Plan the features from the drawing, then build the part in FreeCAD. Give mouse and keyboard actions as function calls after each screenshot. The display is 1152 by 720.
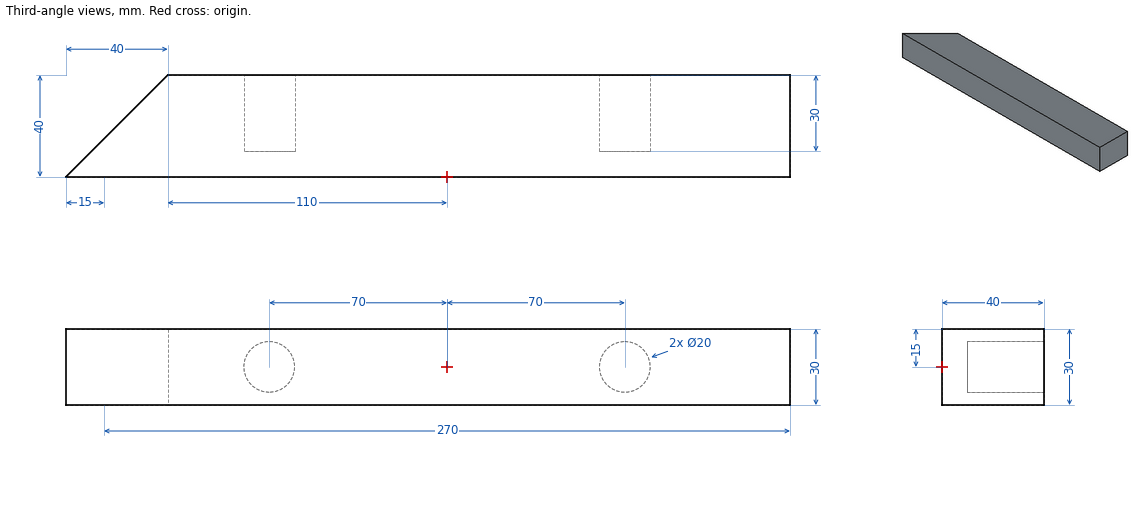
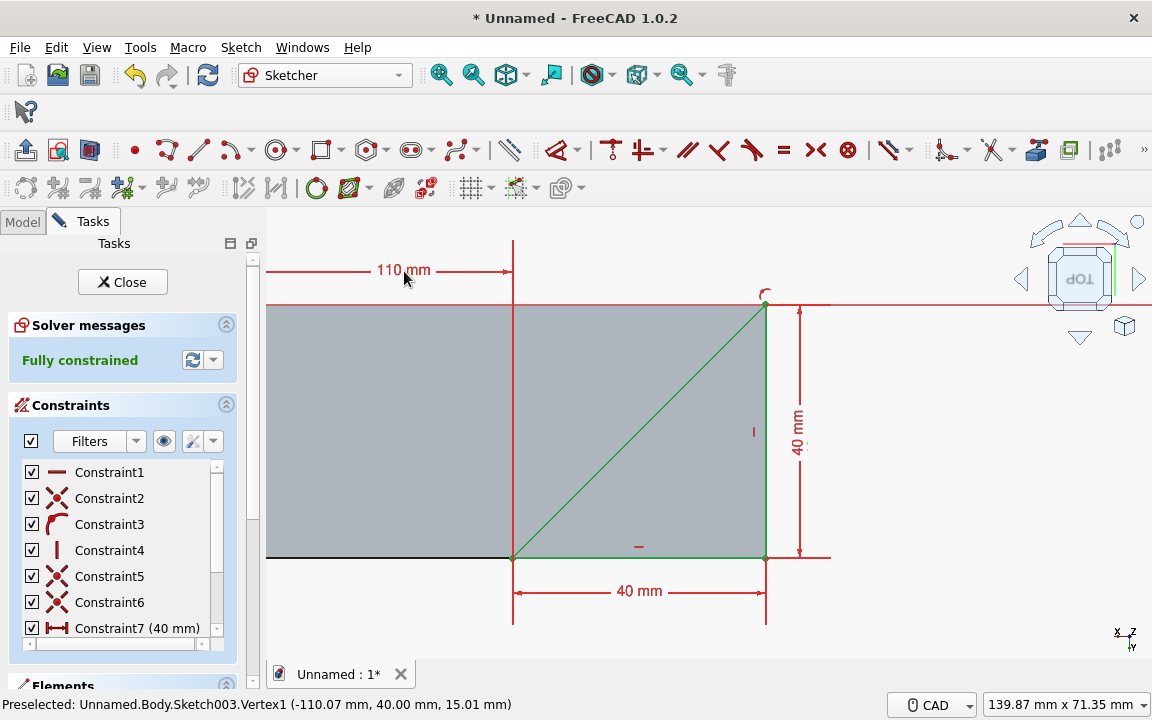
click(123, 282)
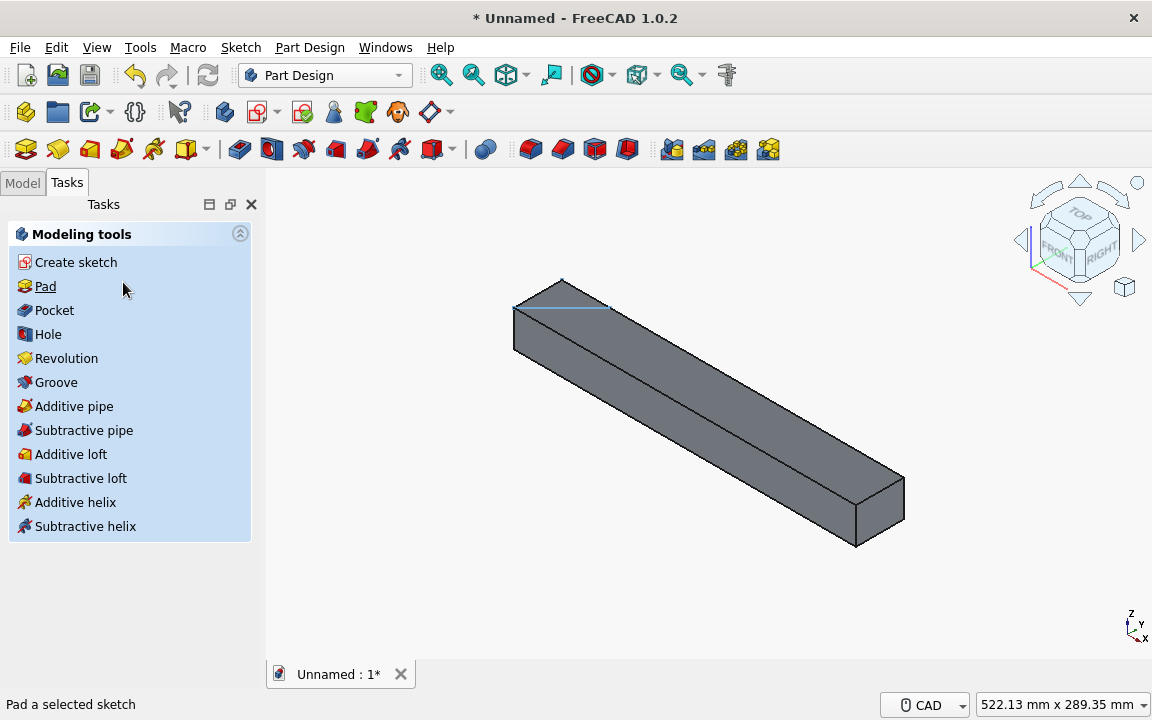
click(240, 150)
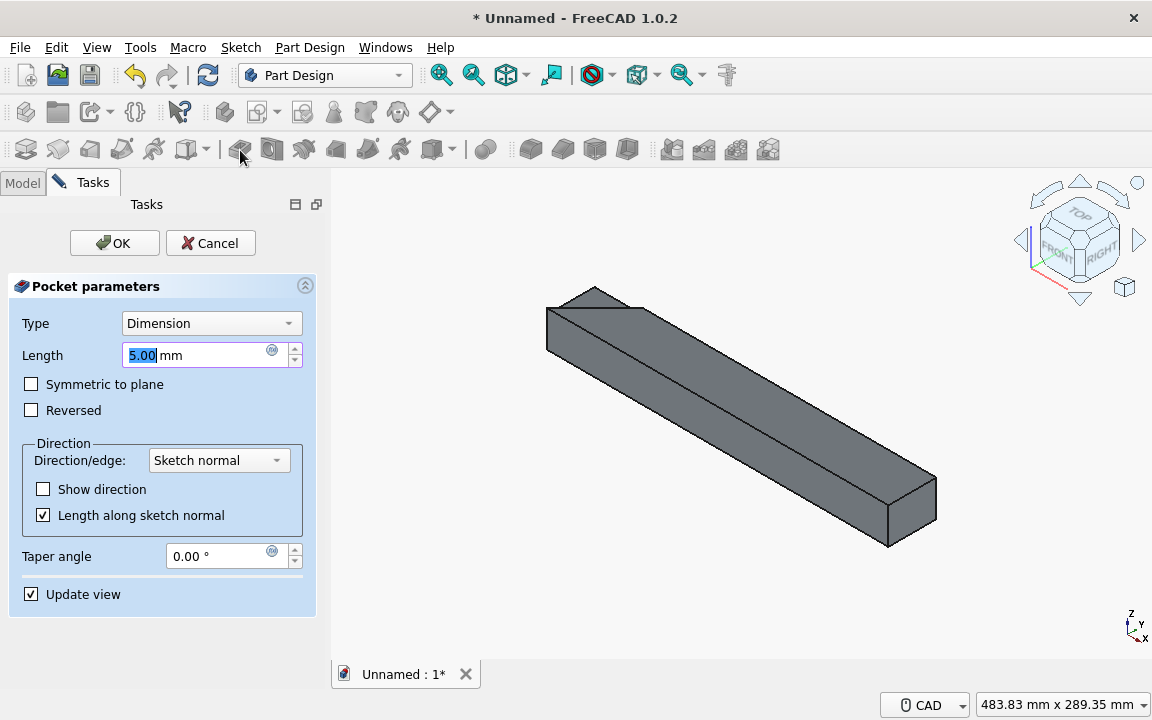
click(212, 324)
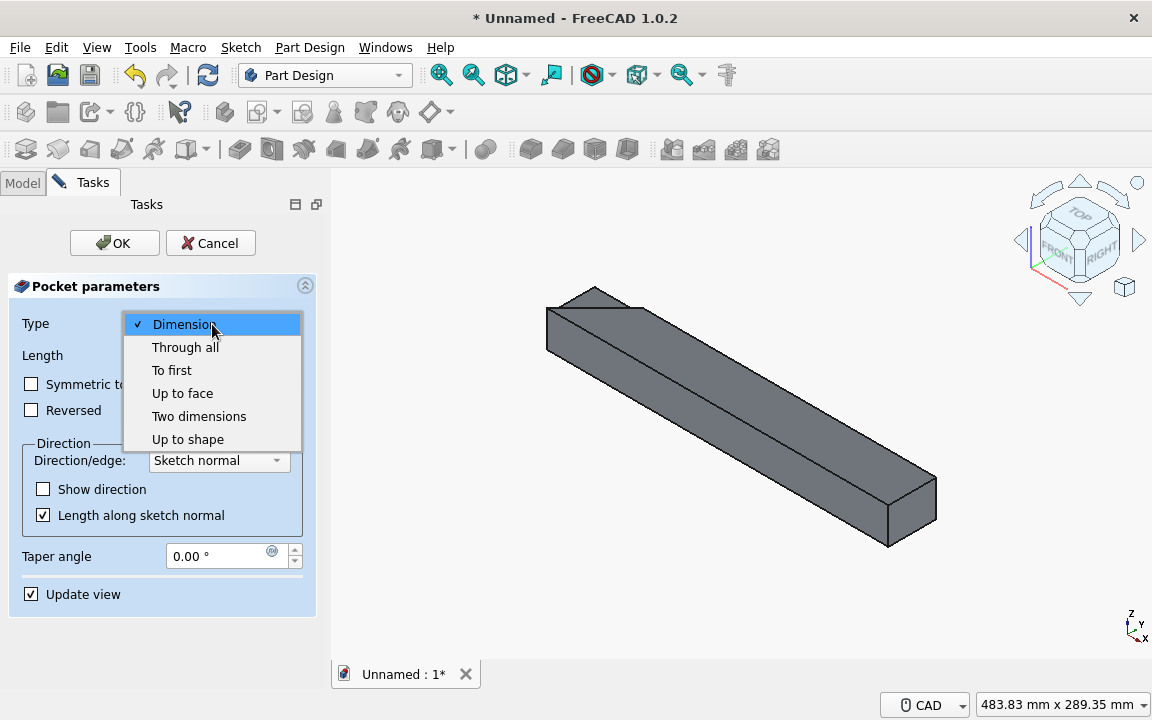
click(212, 348)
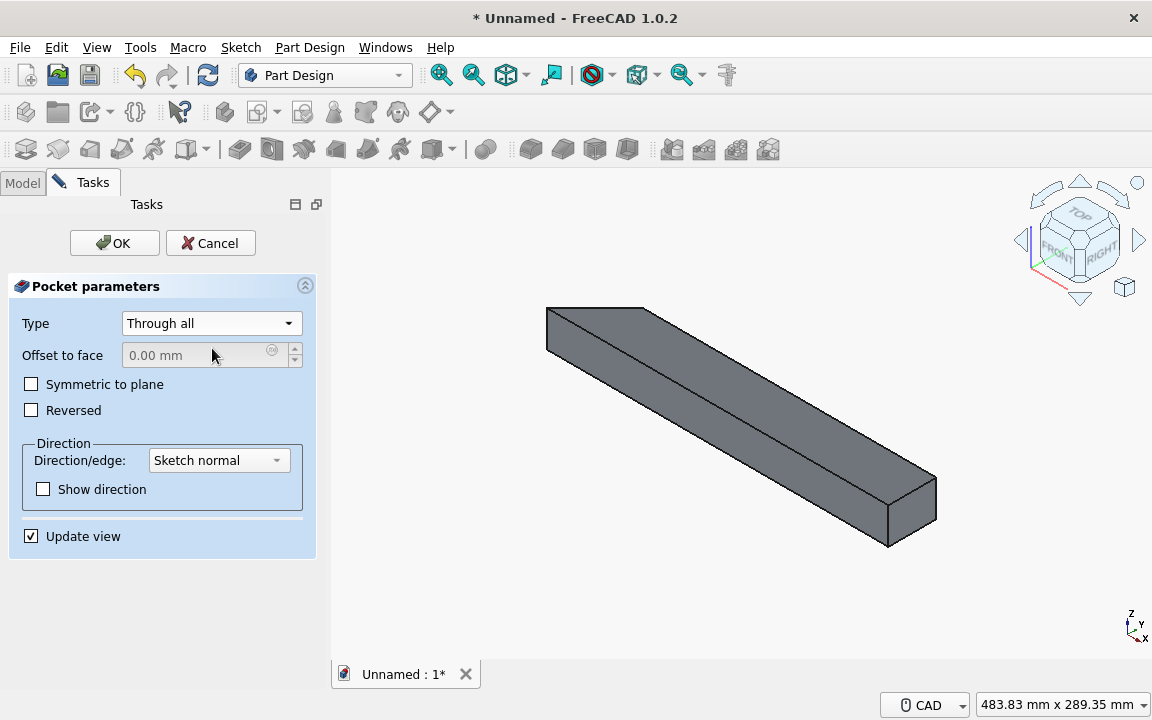
click(115, 243)